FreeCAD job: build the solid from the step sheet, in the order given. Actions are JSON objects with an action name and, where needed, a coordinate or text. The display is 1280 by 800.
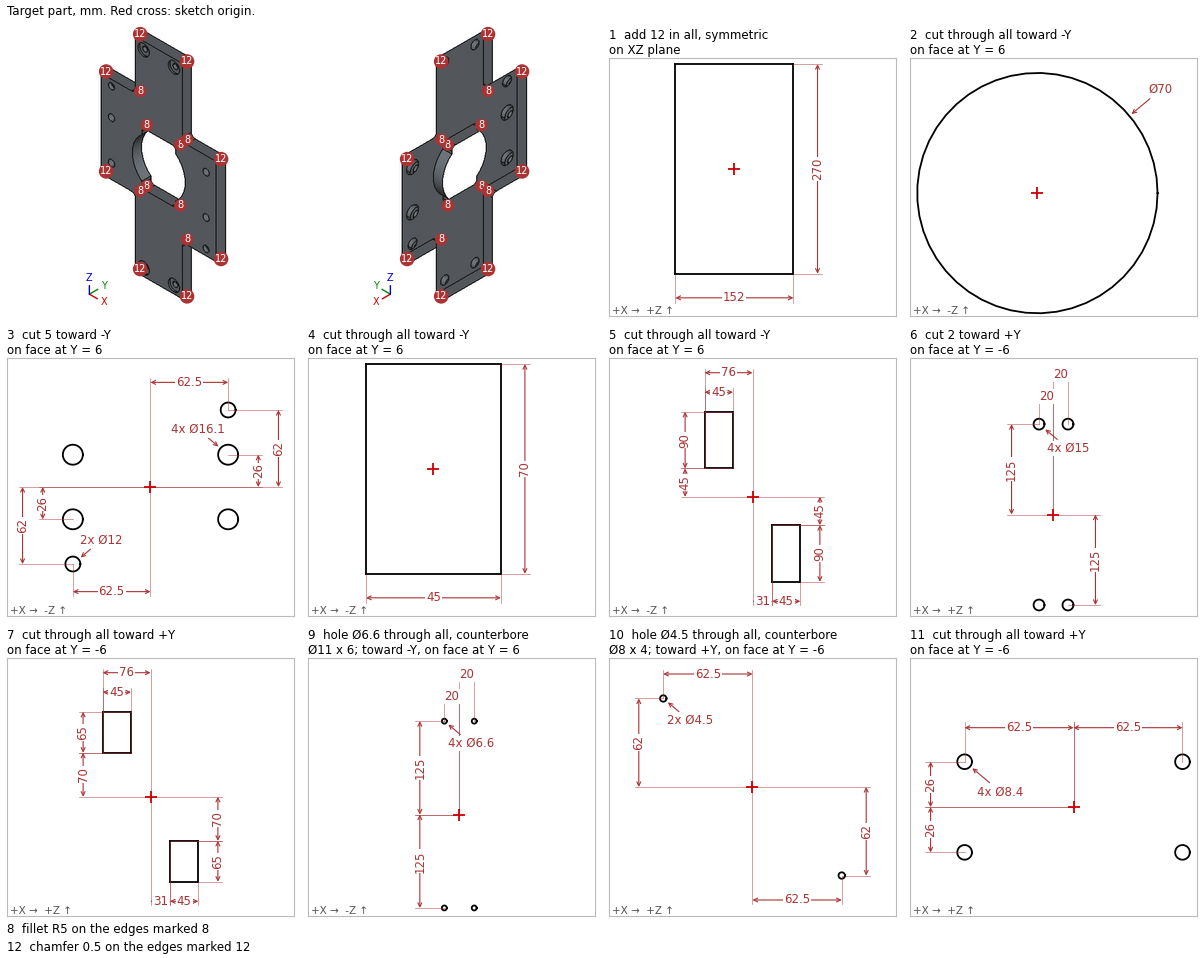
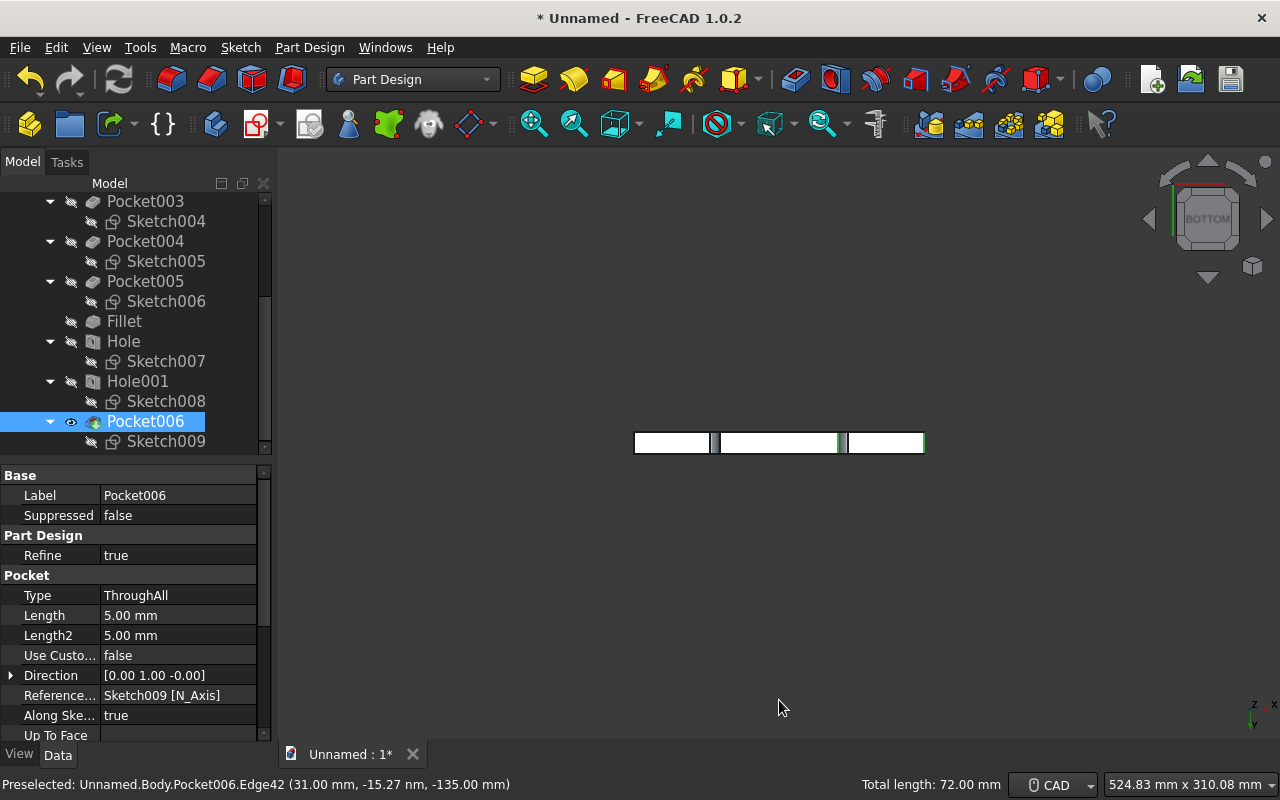
{"action": "left_click", "coordinate": [634, 442], "text": "ctrl"}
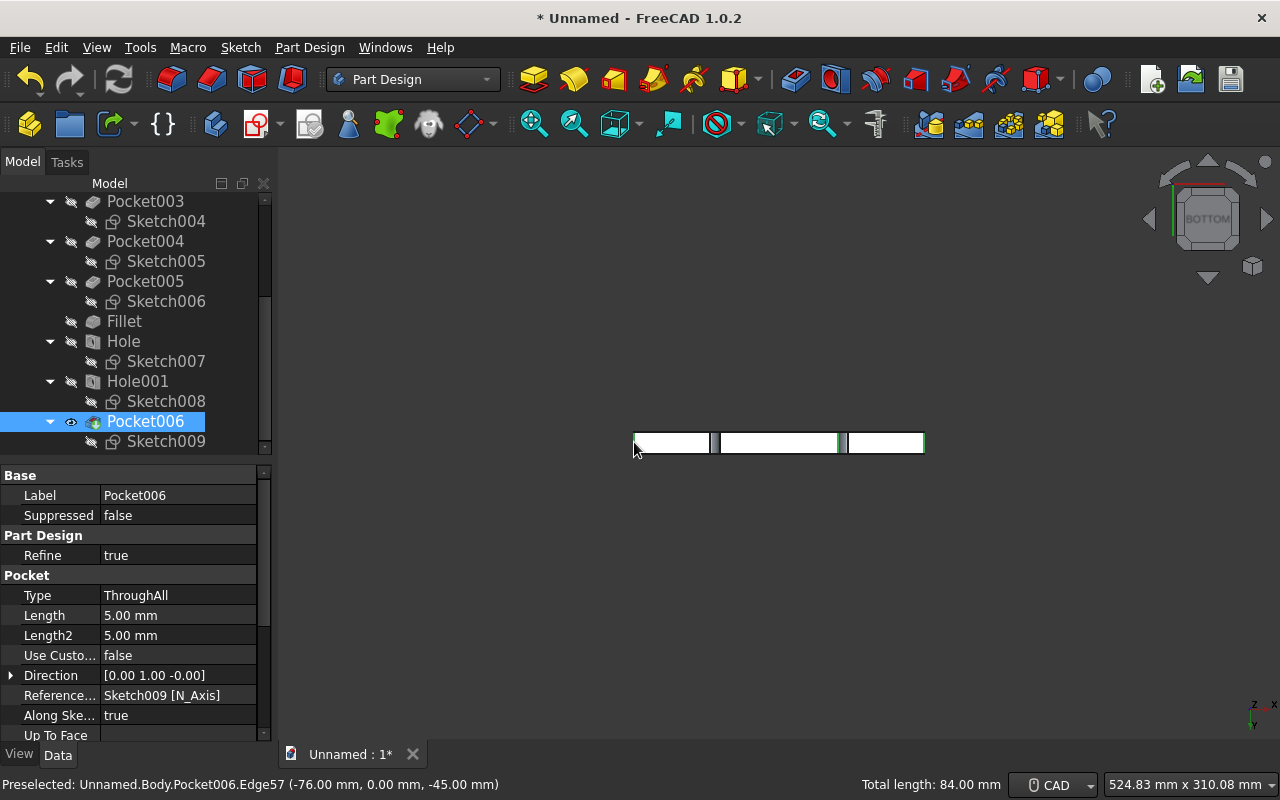
{"action": "left_click", "coordinate": [720, 442], "text": "ctrl"}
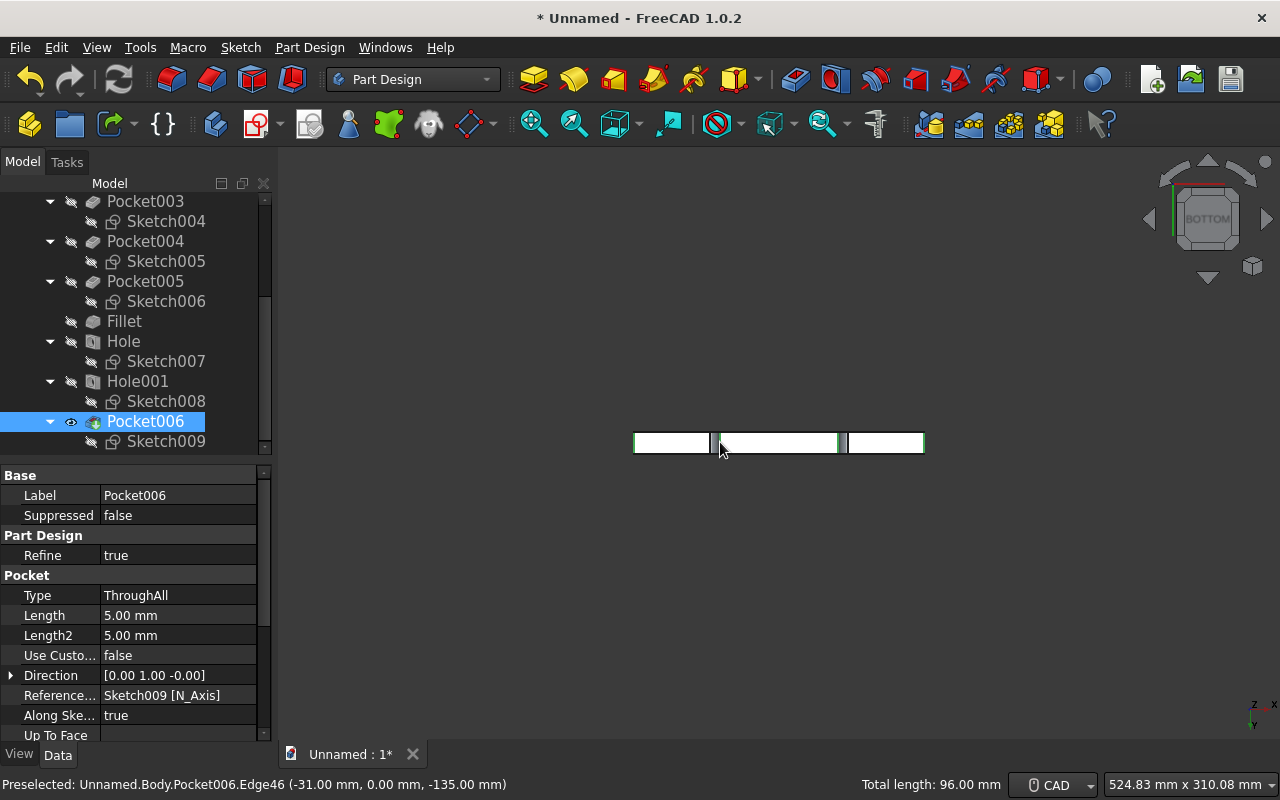
{"action": "left_click", "coordinate": [212, 80]}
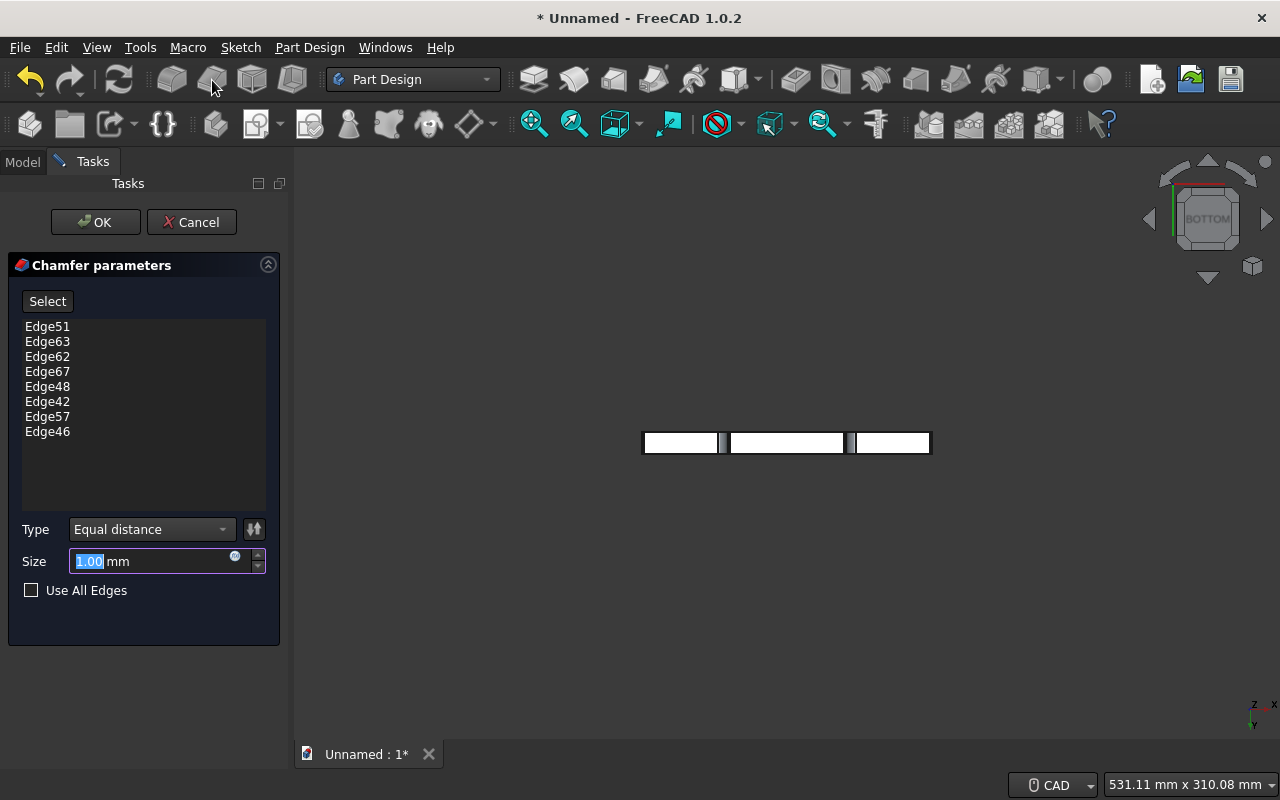
{"action": "type", "text": "0.5"}
{"action": "key", "text": "Tab"}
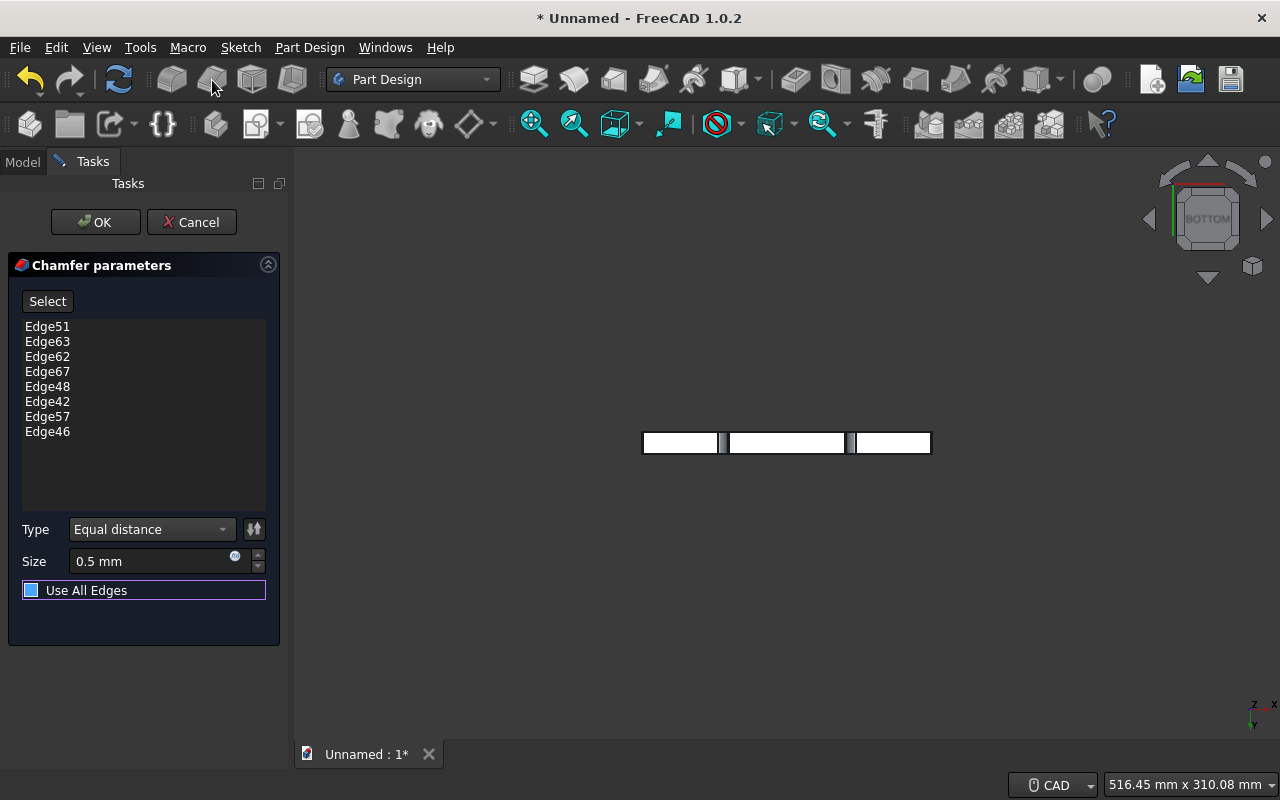
{"action": "left_click", "coordinate": [96, 222]}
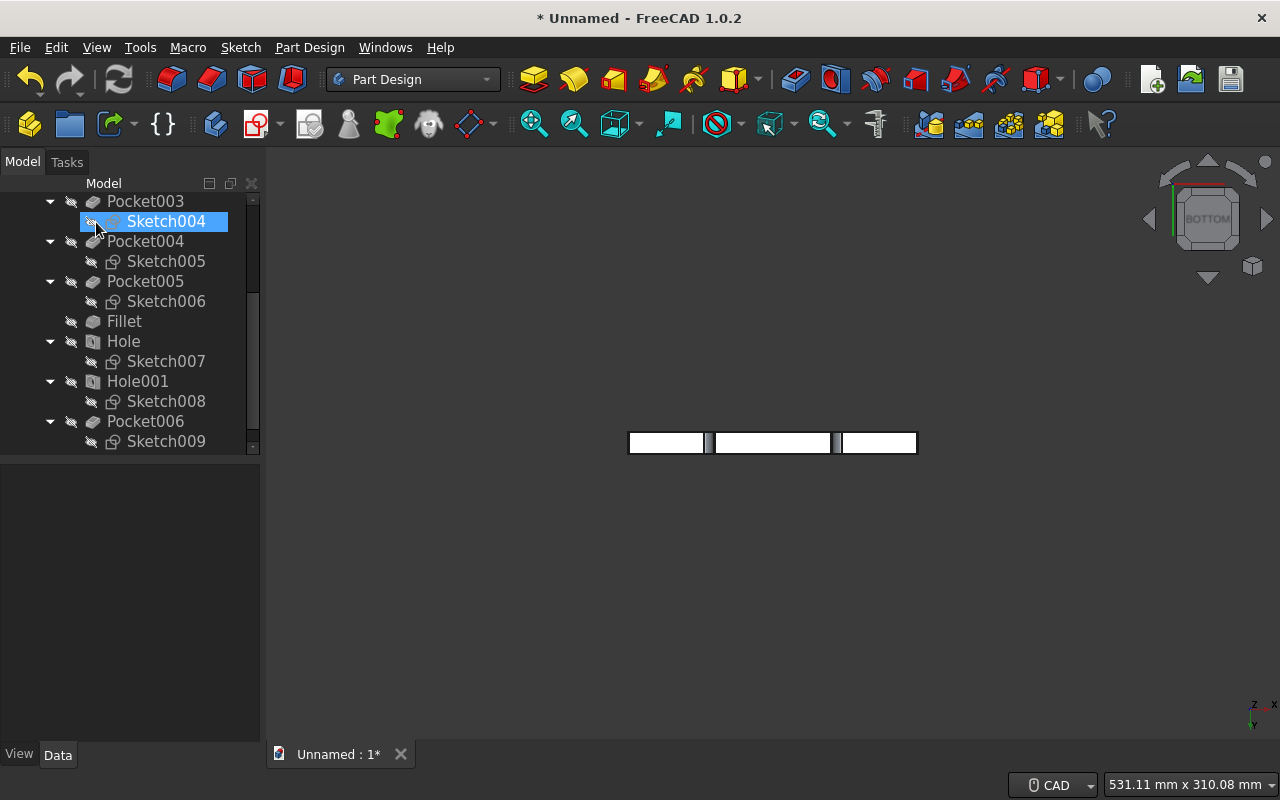
{"action": "key", "text": "0"}